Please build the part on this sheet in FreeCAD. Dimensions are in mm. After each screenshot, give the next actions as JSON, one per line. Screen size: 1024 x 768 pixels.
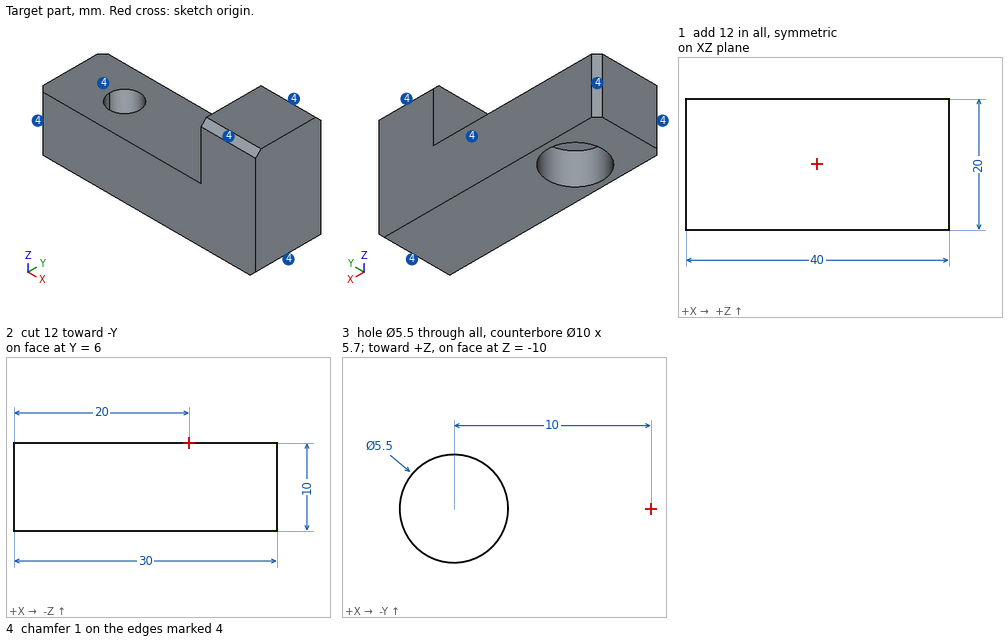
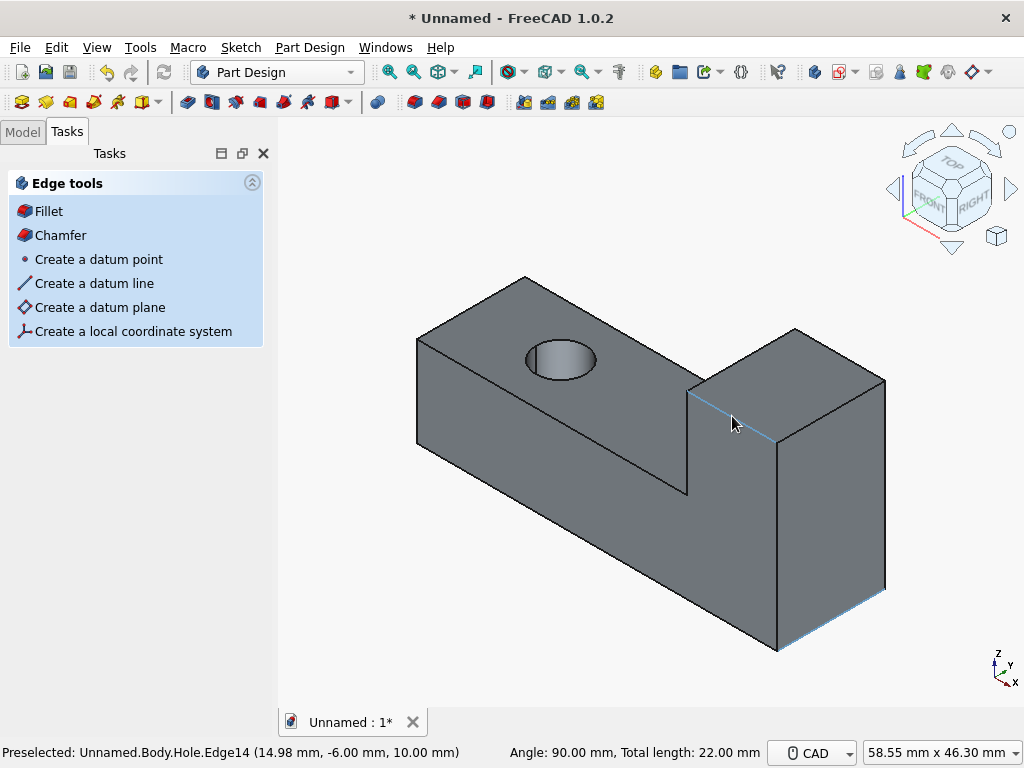
{"action": "key", "text": "2"}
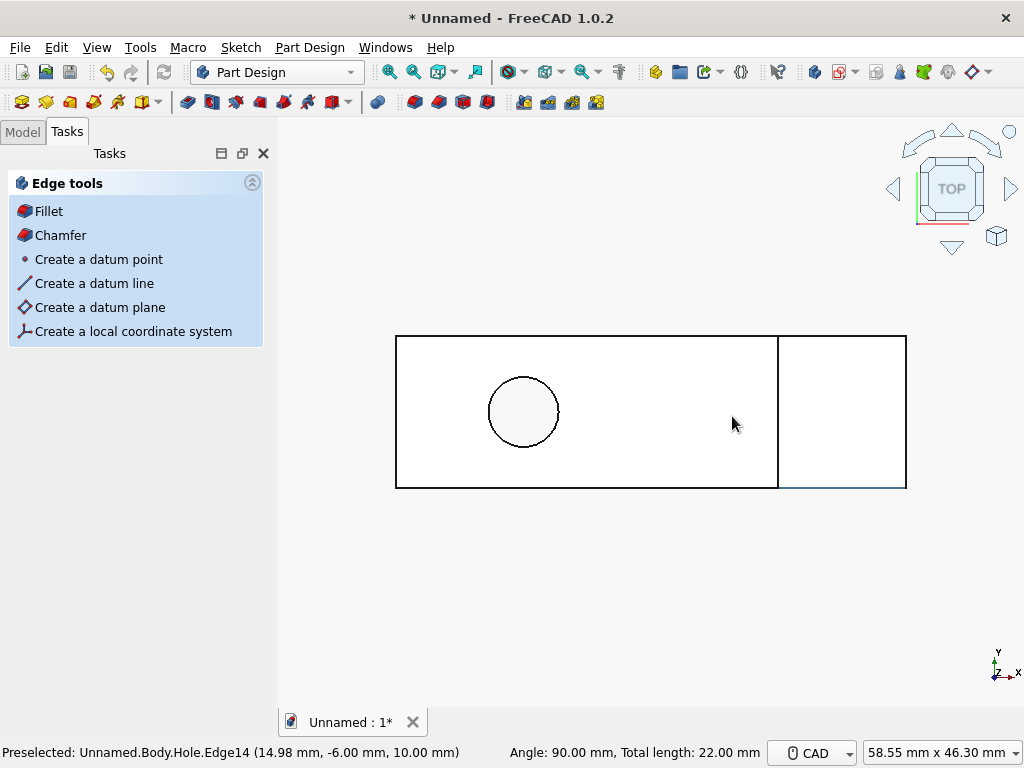
{"action": "left_click", "coordinate": [842, 335], "text": "ctrl"}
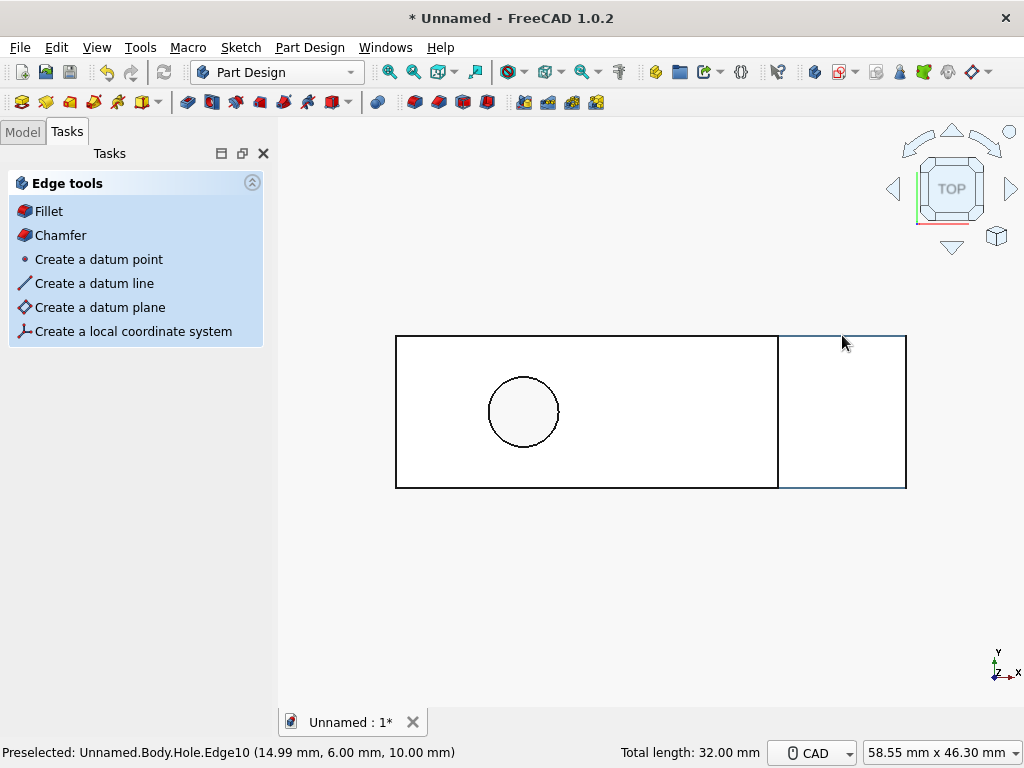
{"action": "key", "text": "1"}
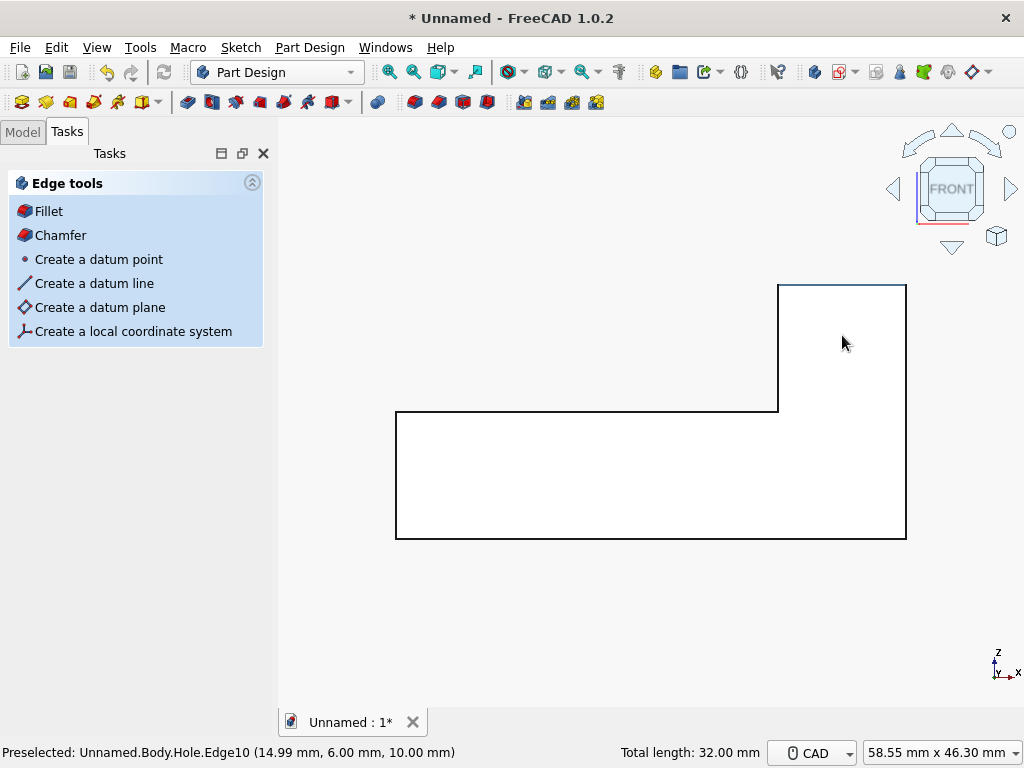
{"action": "left_click", "coordinate": [396, 475], "text": "ctrl"}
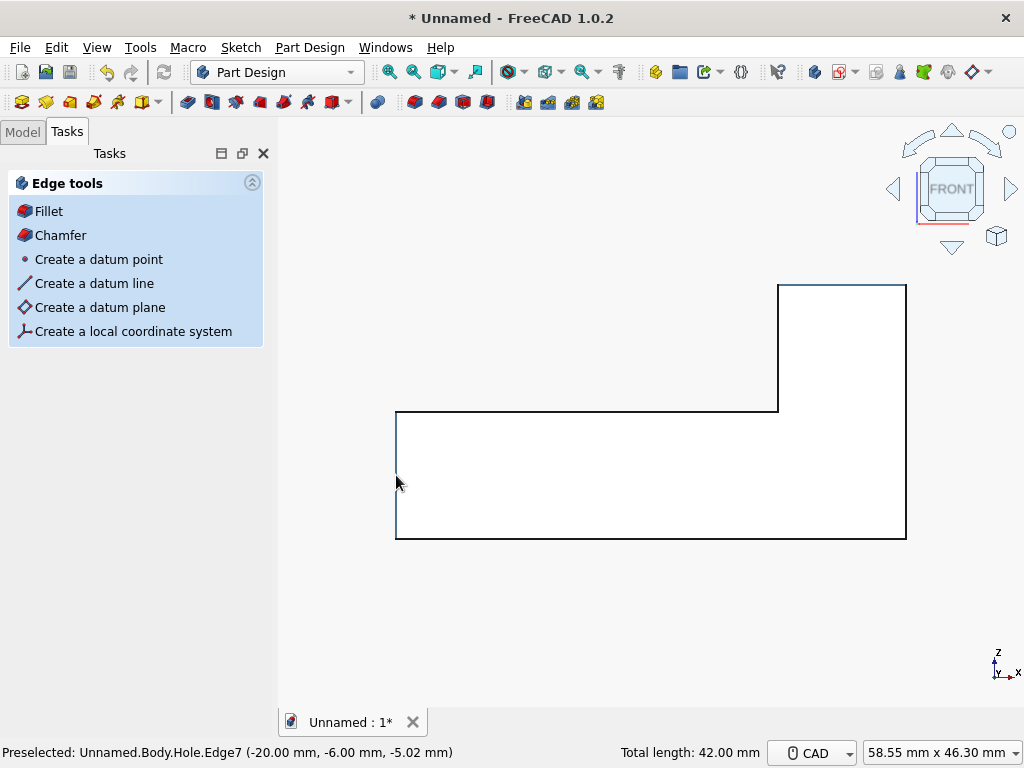
{"action": "key", "text": "3"}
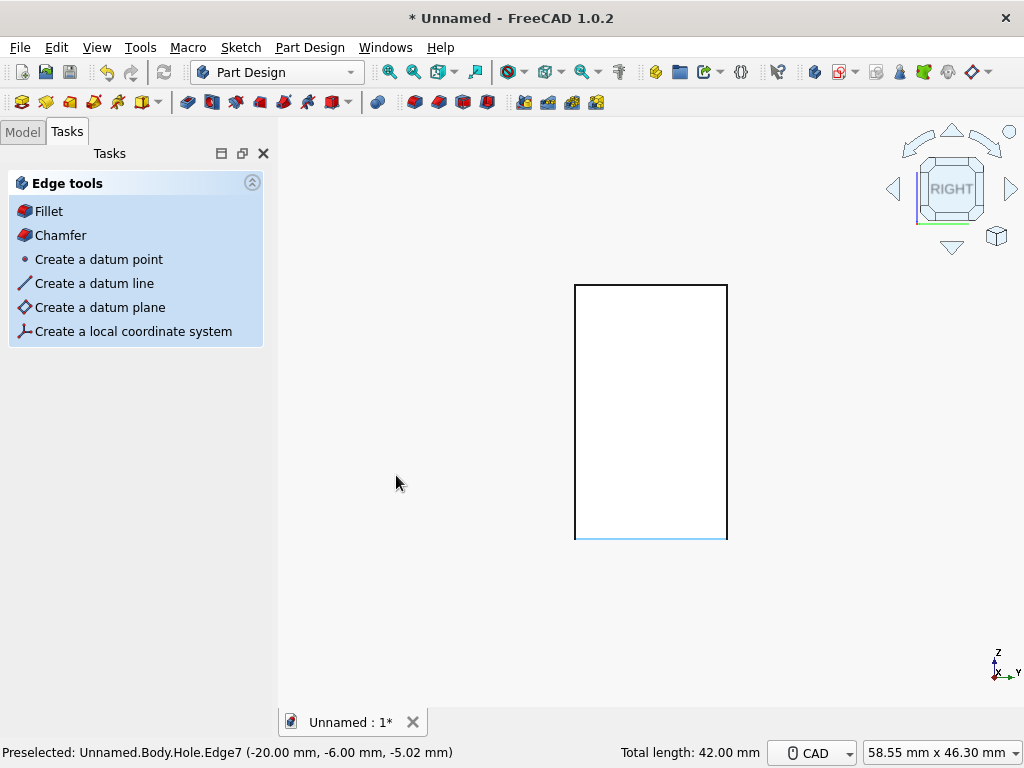
{"action": "key", "text": "v f"}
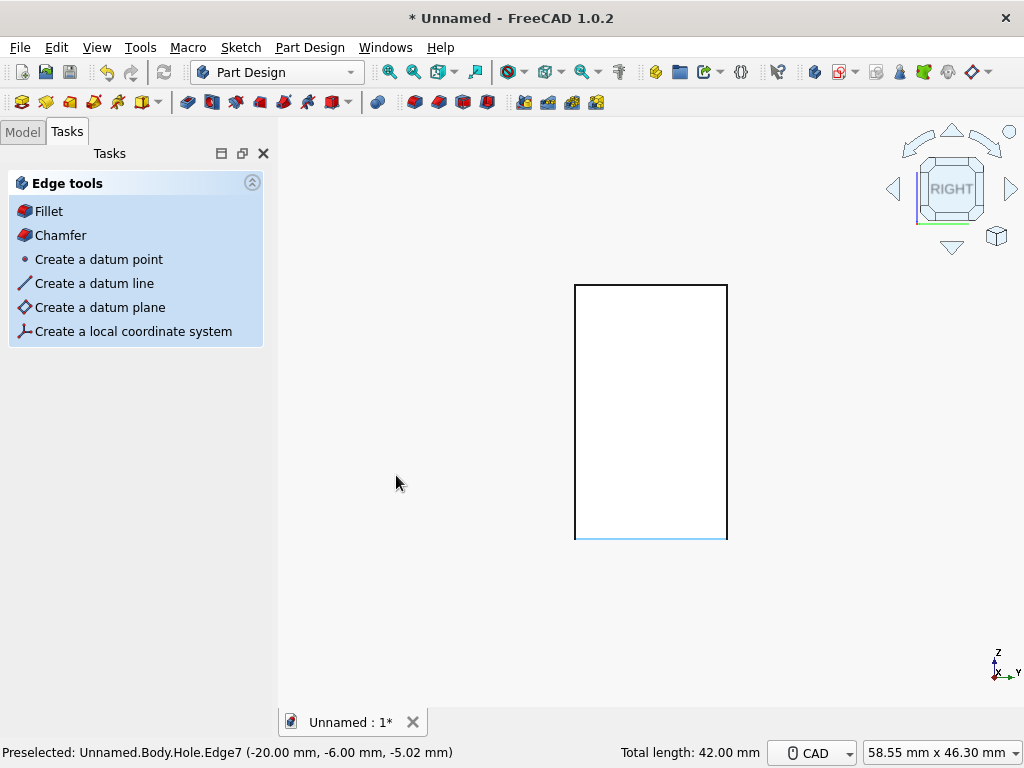
{"action": "key", "text": "5"}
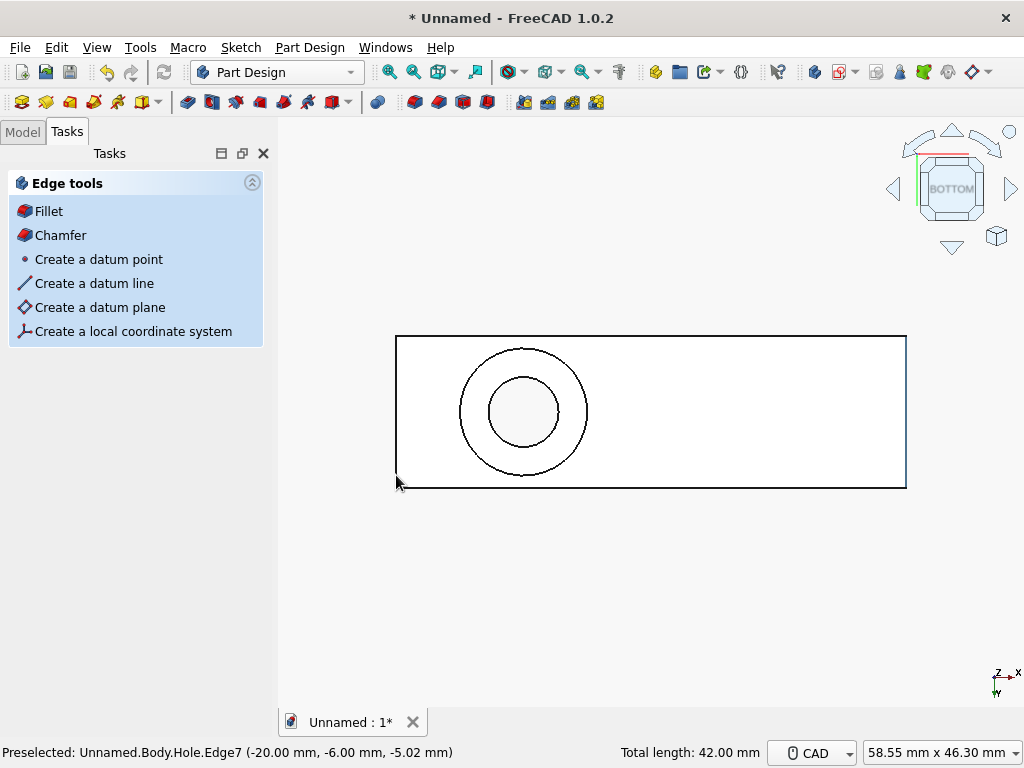
{"action": "key", "text": "4"}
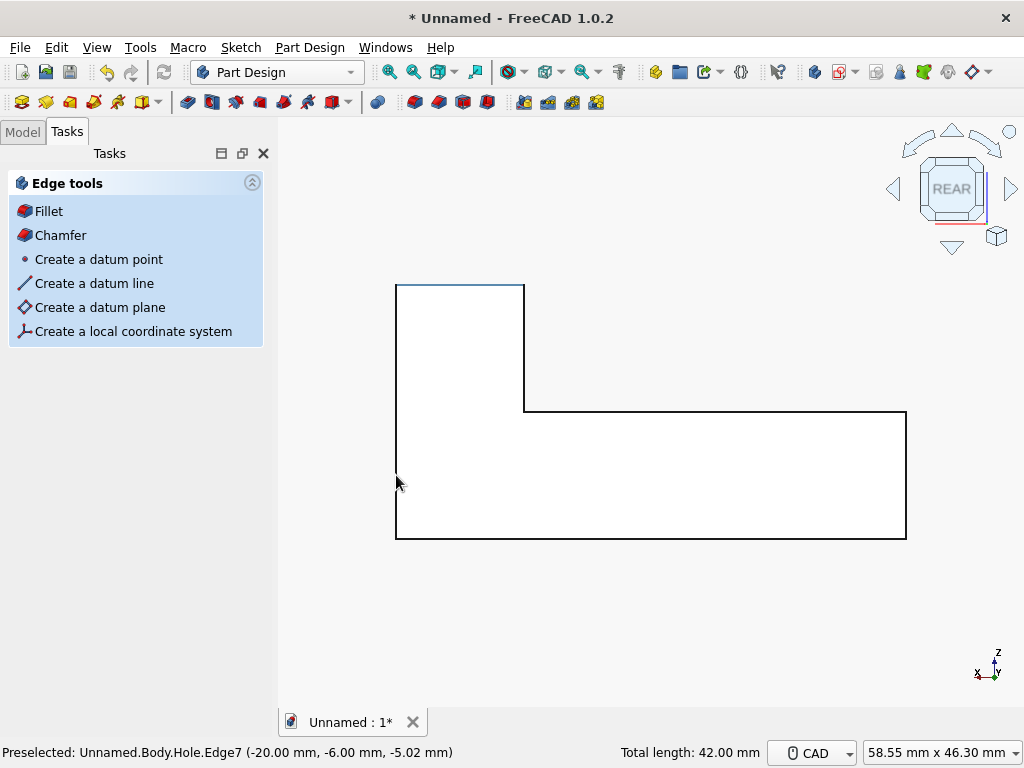
{"action": "left_click", "coordinate": [906, 475], "text": "ctrl"}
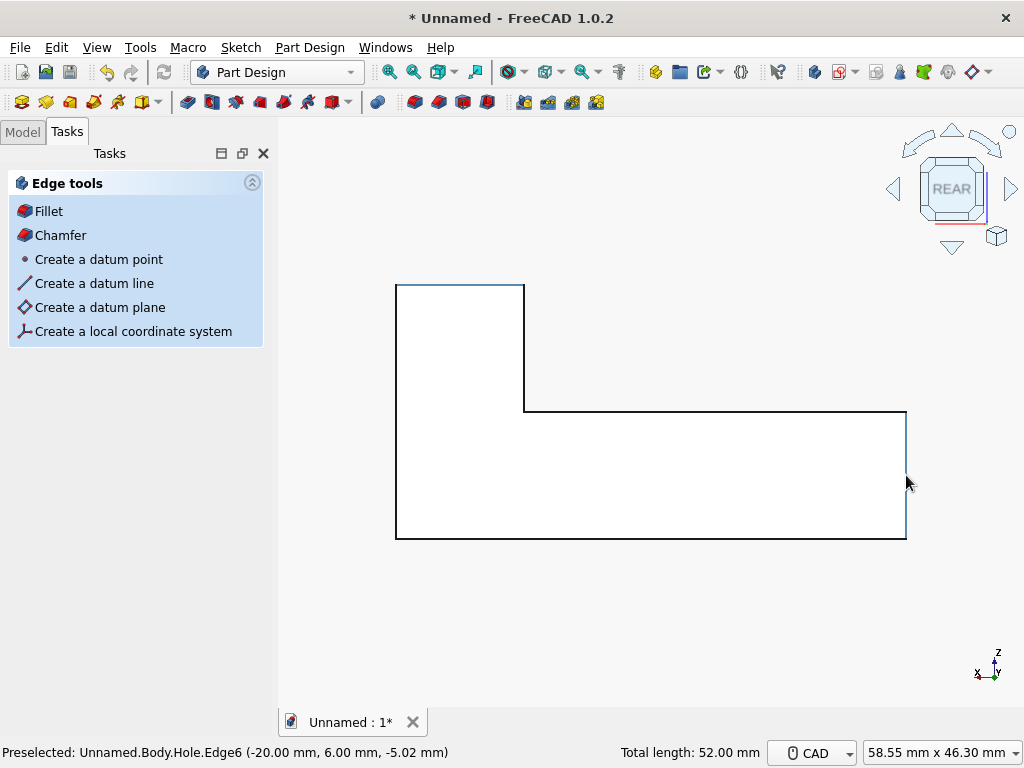
{"action": "left_click", "coordinate": [440, 102]}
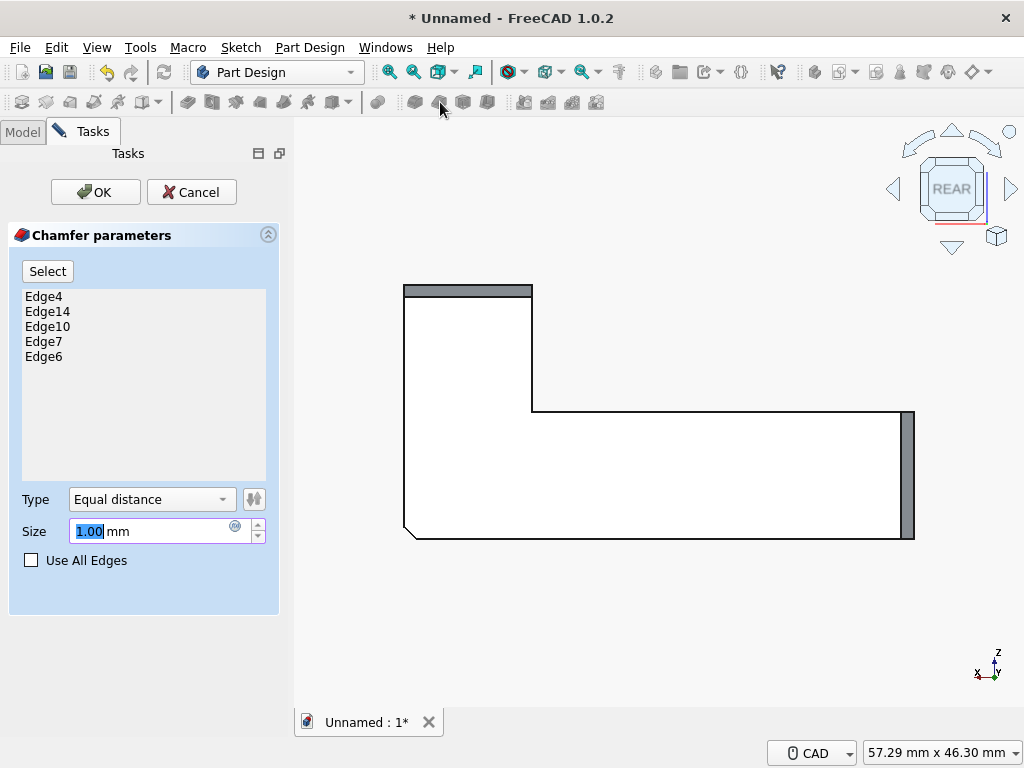
{"action": "type", "text": "1"}
{"action": "key", "text": "Tab"}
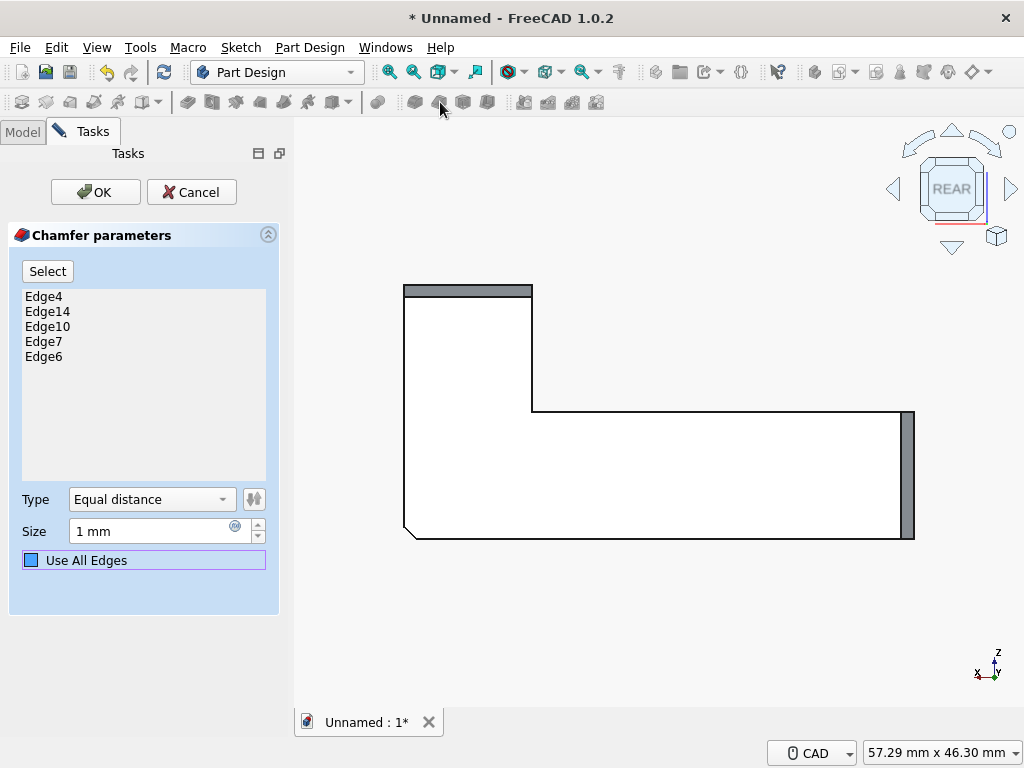
{"action": "left_click", "coordinate": [96, 192]}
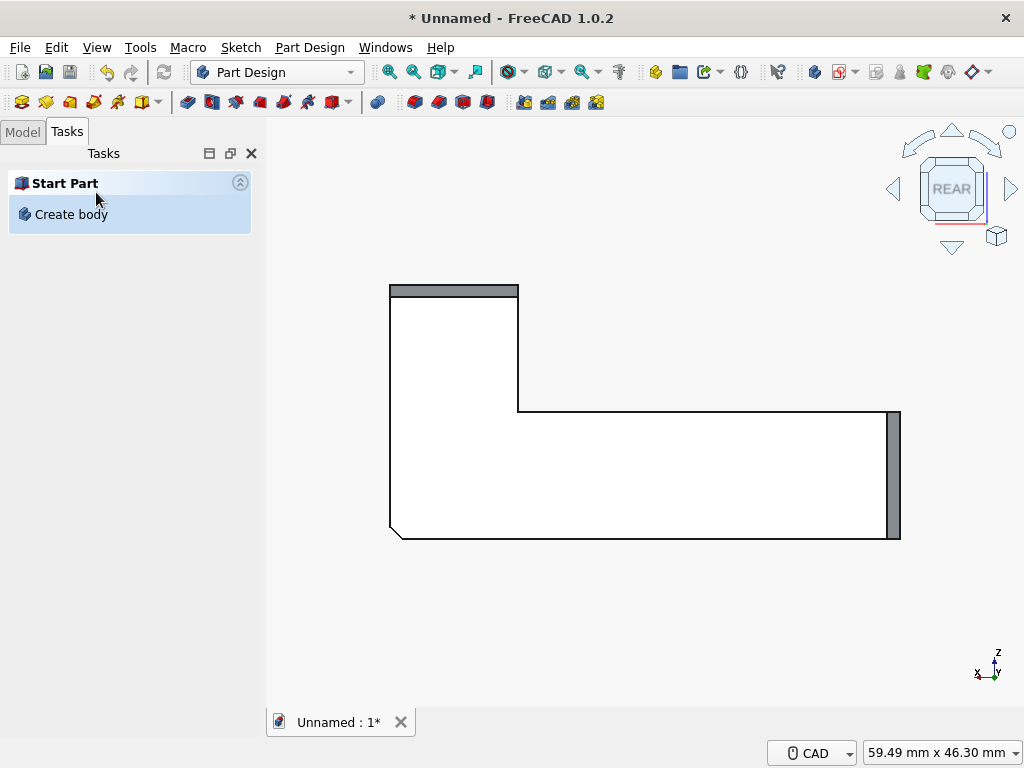
{"action": "key", "text": "0"}